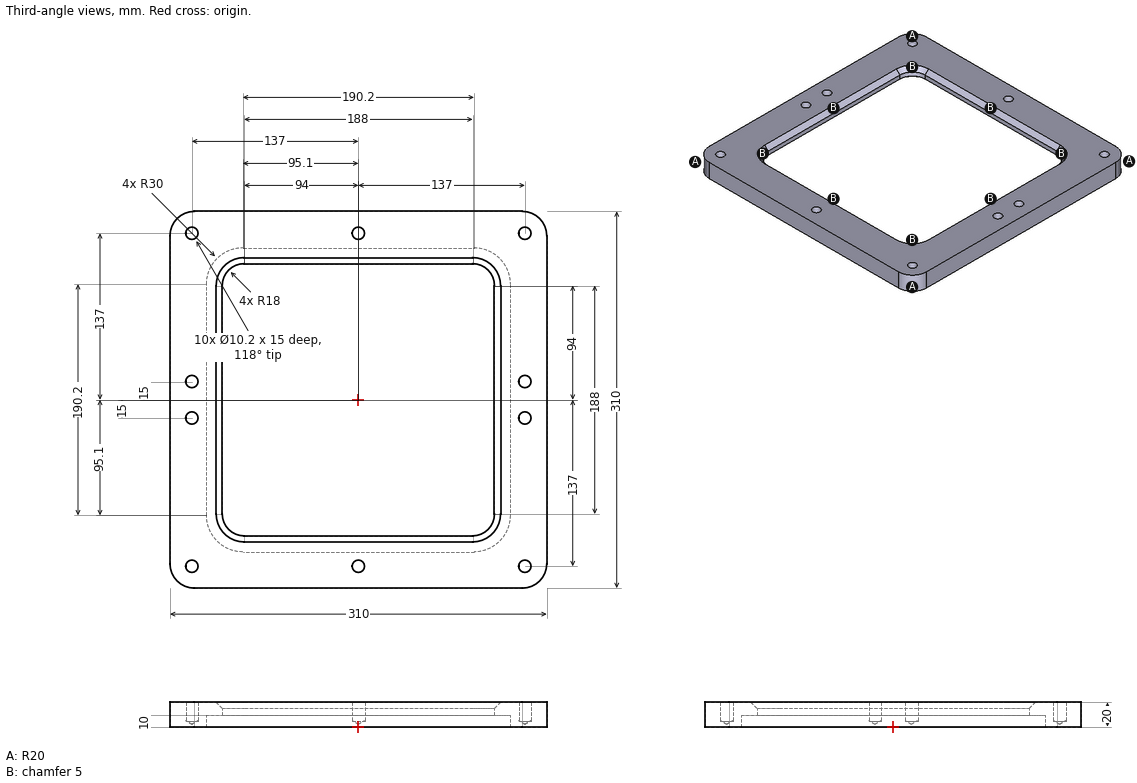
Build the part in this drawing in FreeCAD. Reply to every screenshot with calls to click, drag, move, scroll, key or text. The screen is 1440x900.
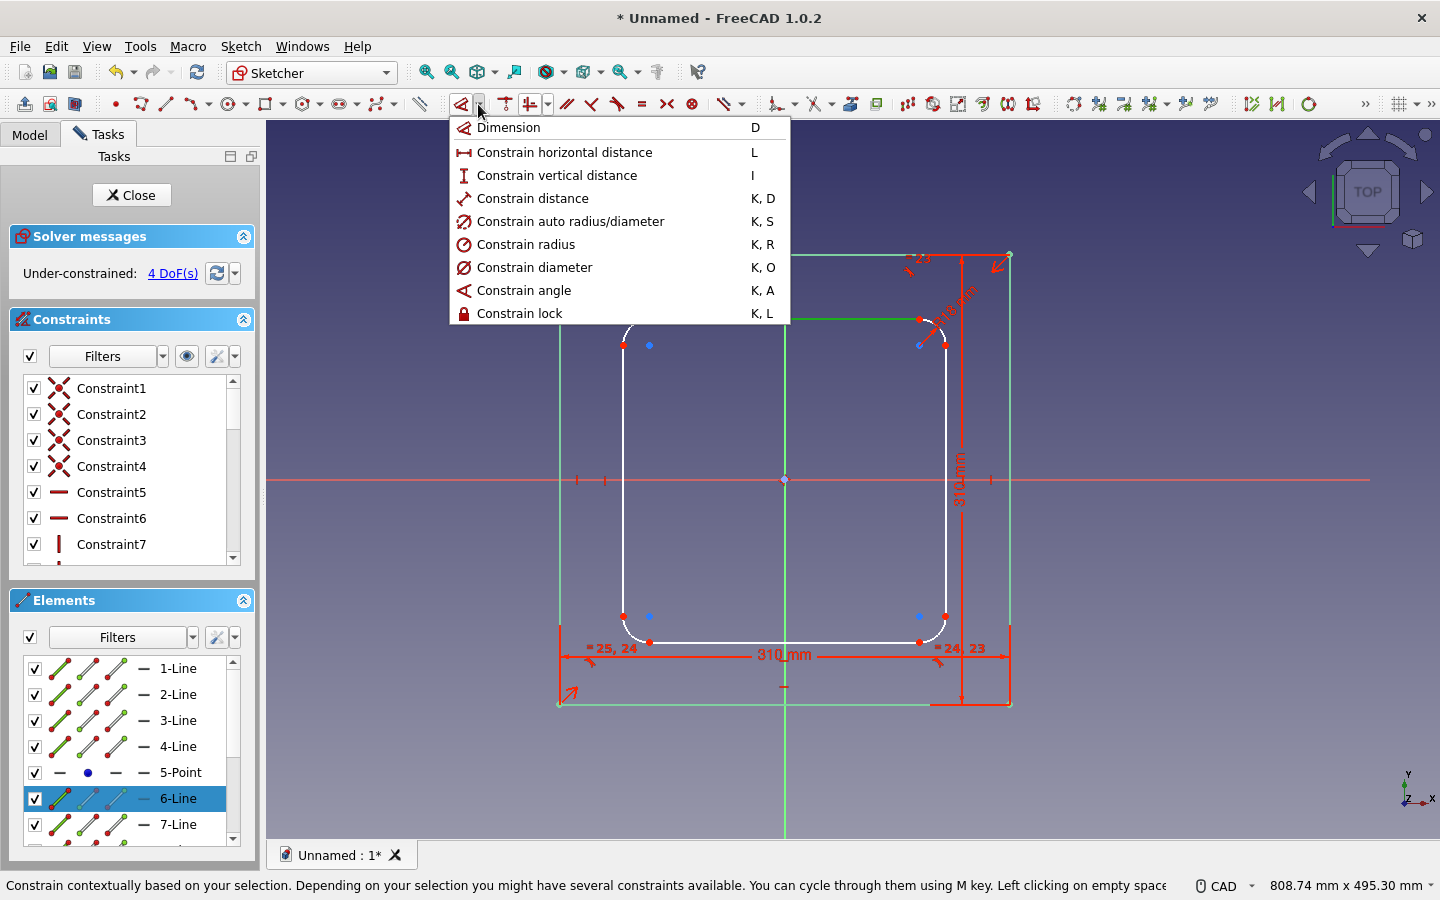
click(620, 152)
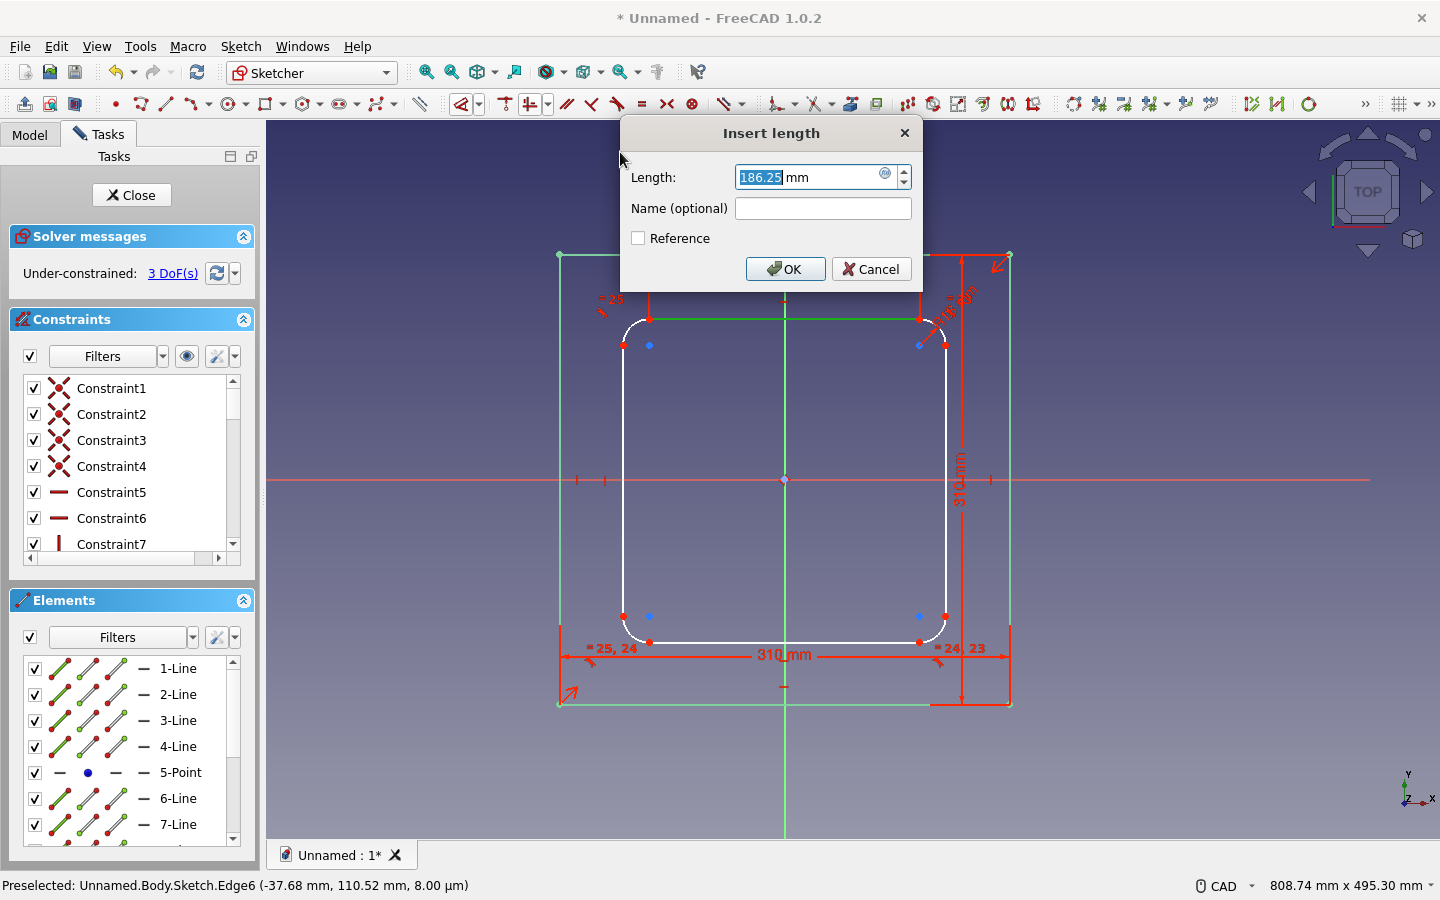
text(188)
key(Return)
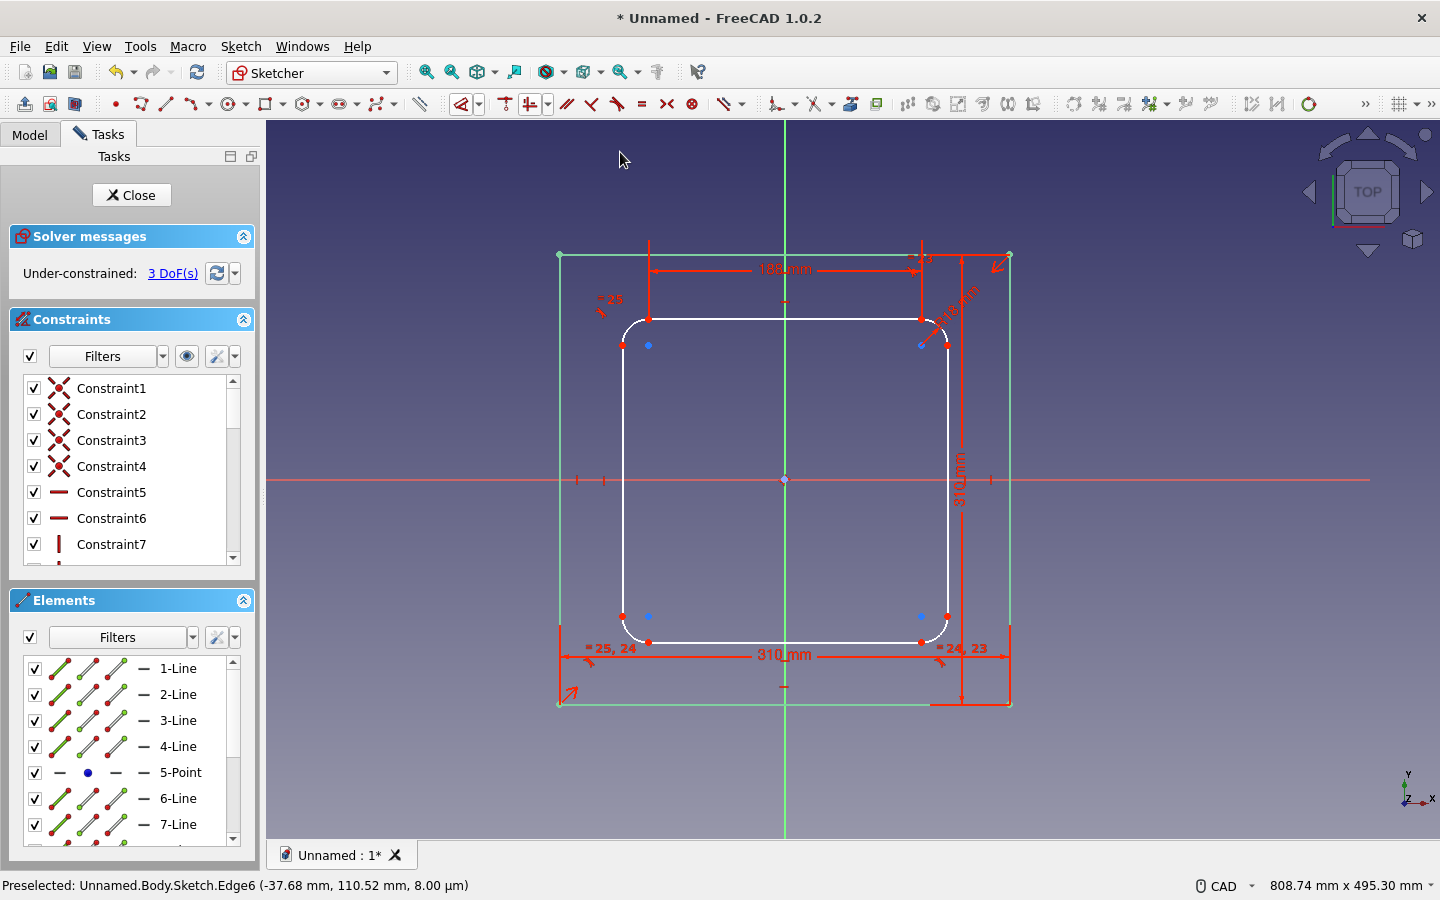
click(948, 427)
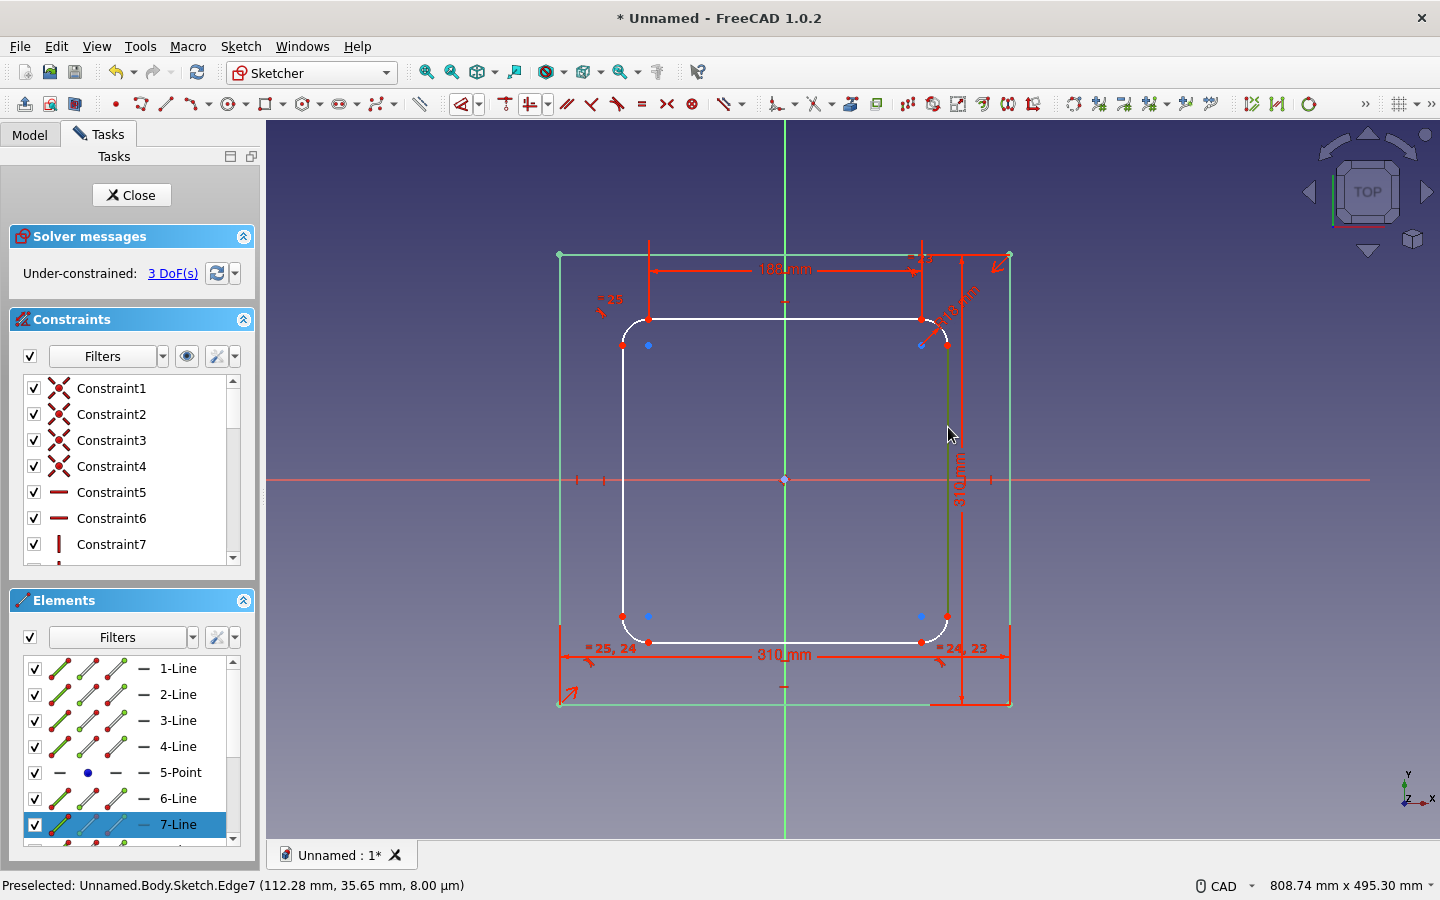
click(478, 104)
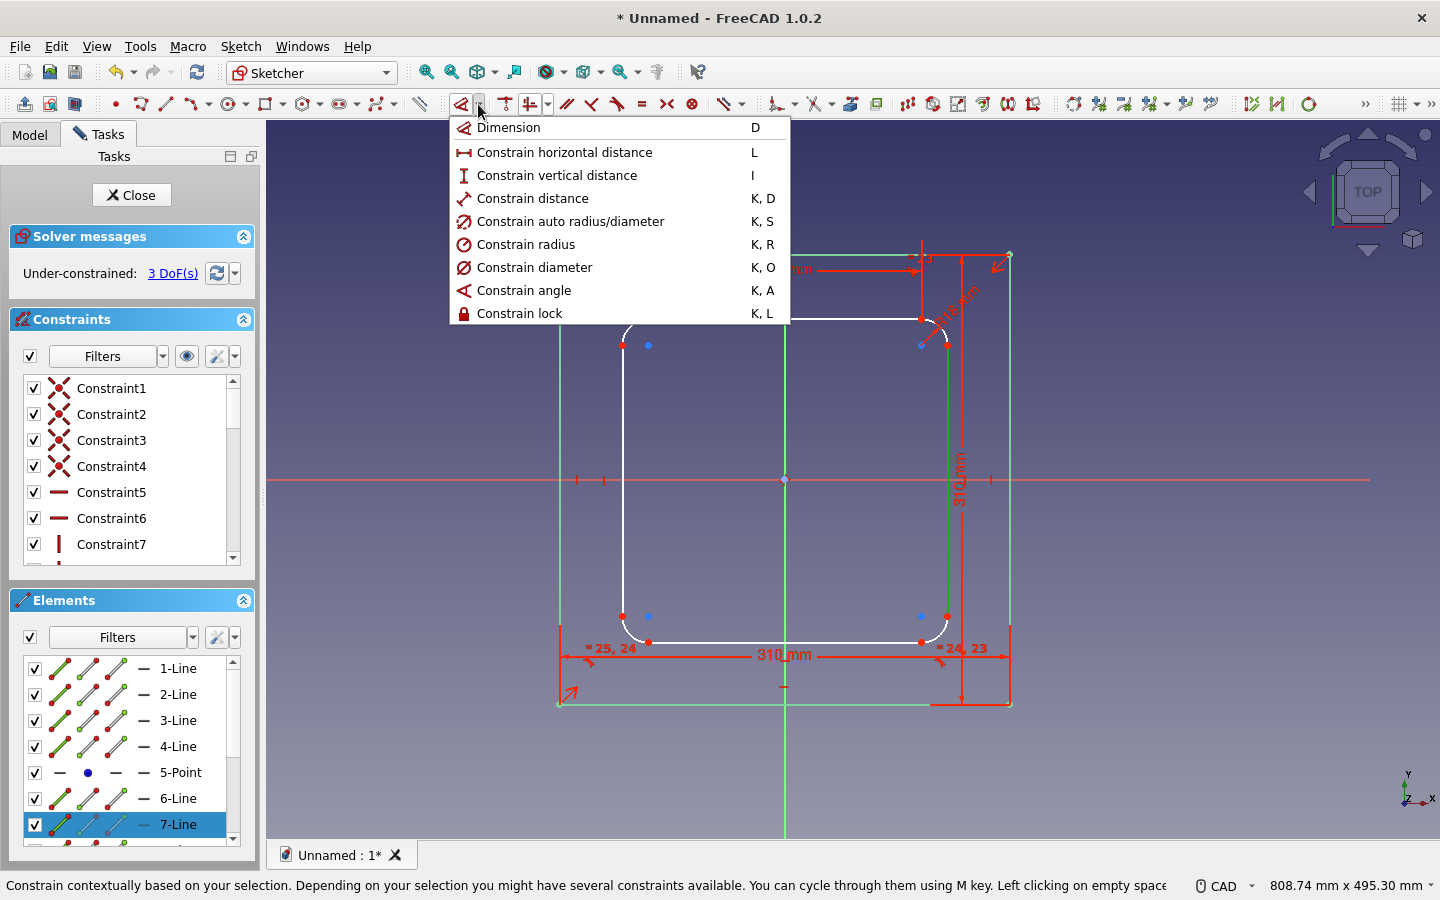
click(620, 176)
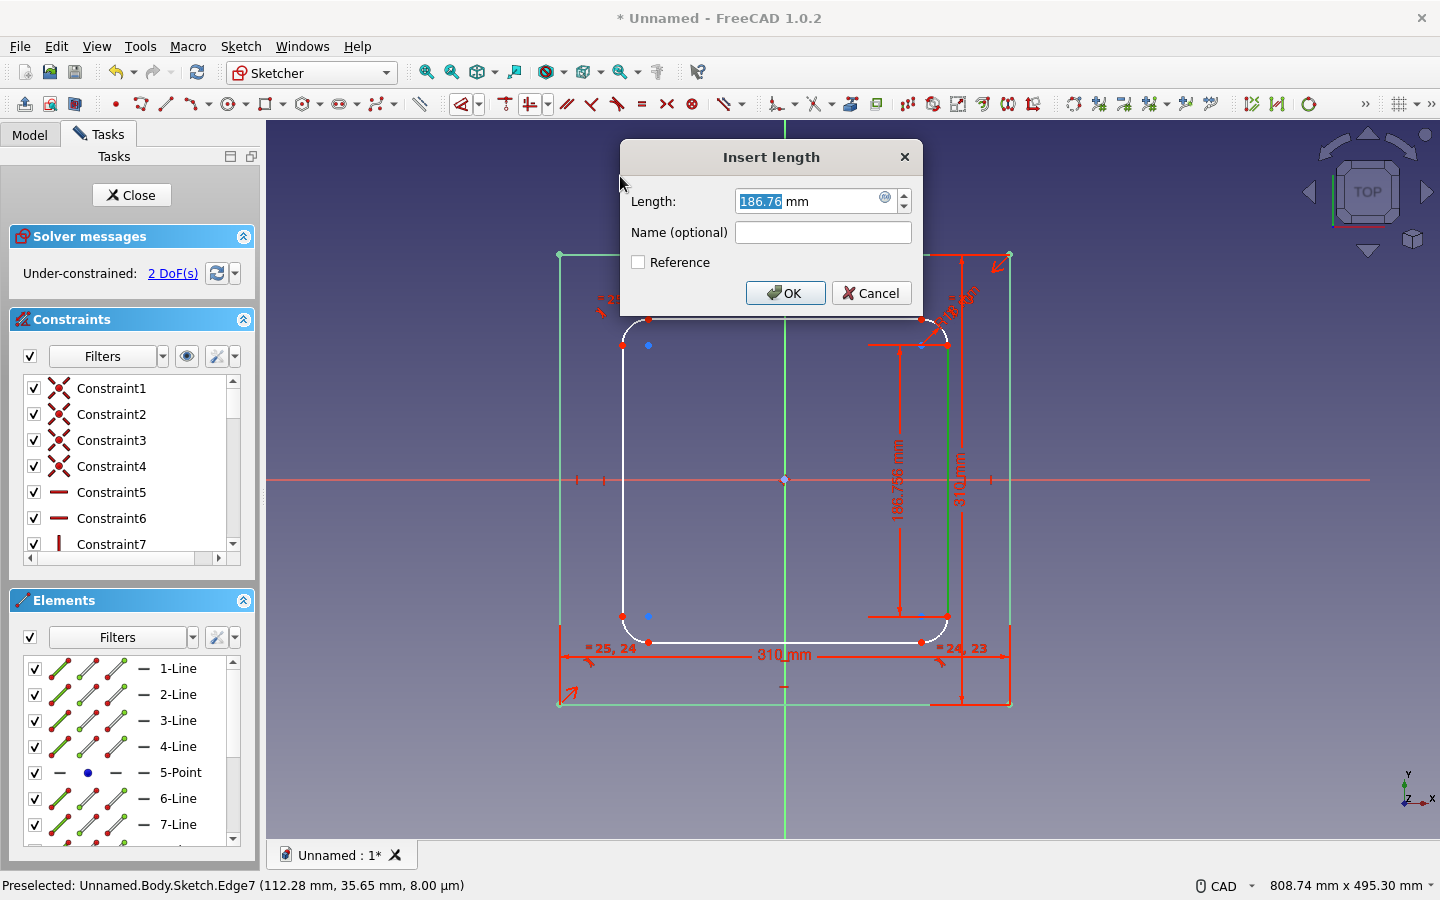
text(188)
key(Return)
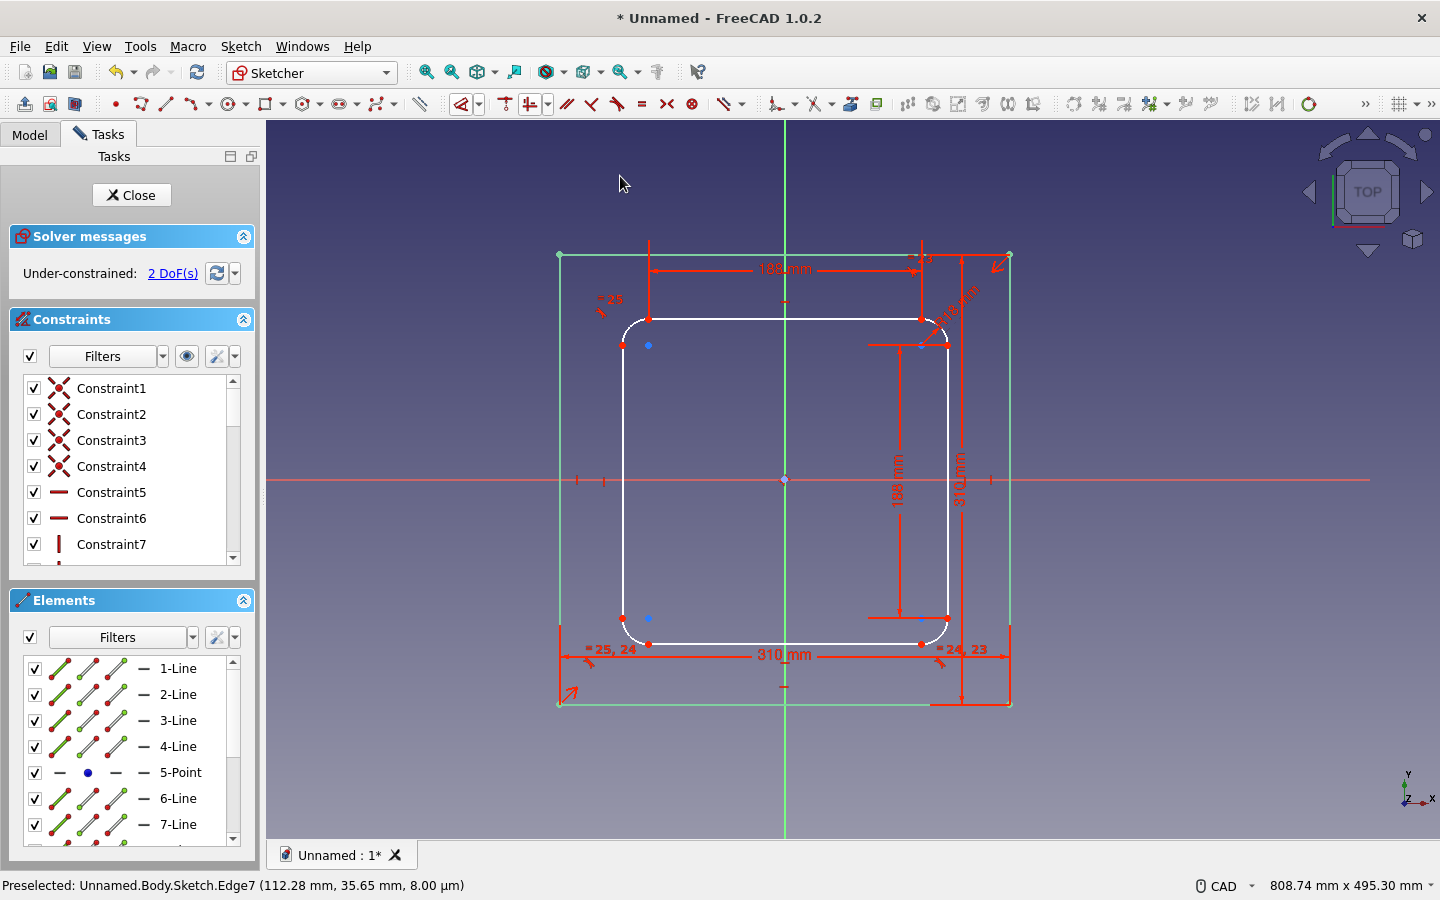
click(649, 319)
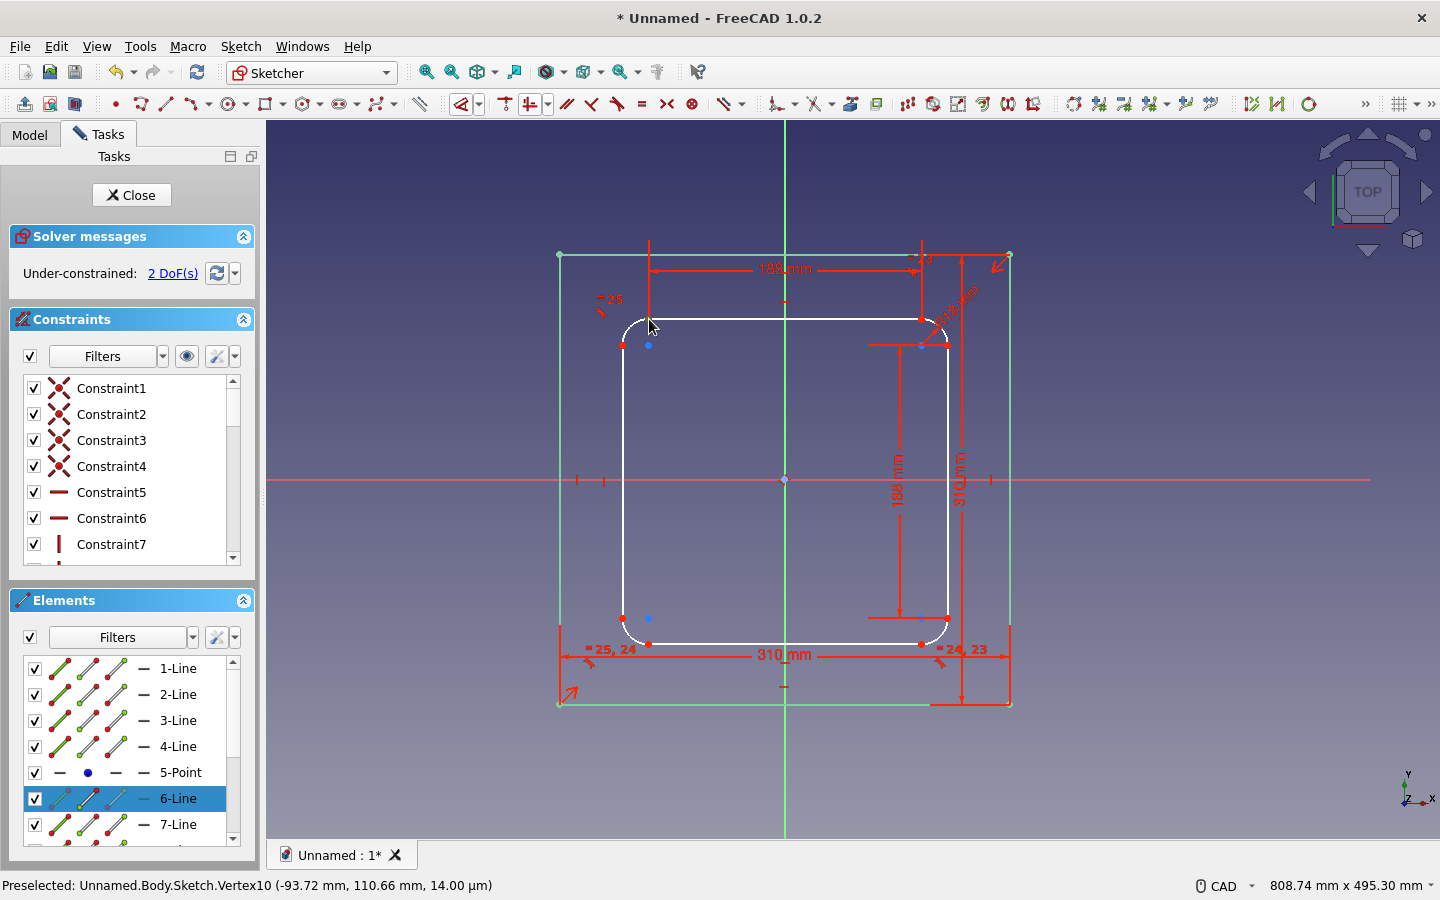
click(478, 104)